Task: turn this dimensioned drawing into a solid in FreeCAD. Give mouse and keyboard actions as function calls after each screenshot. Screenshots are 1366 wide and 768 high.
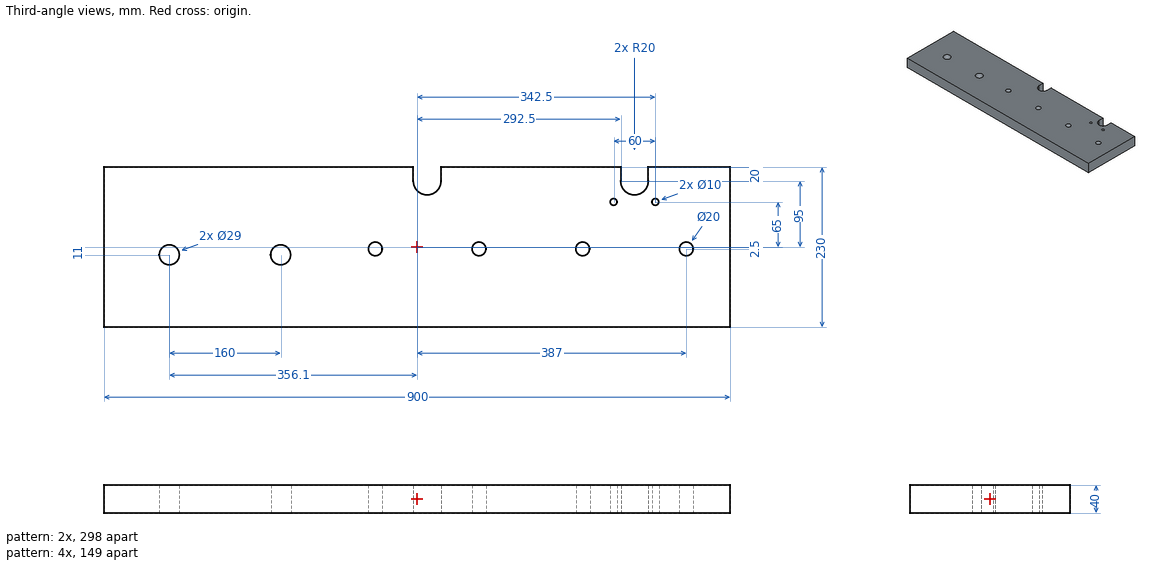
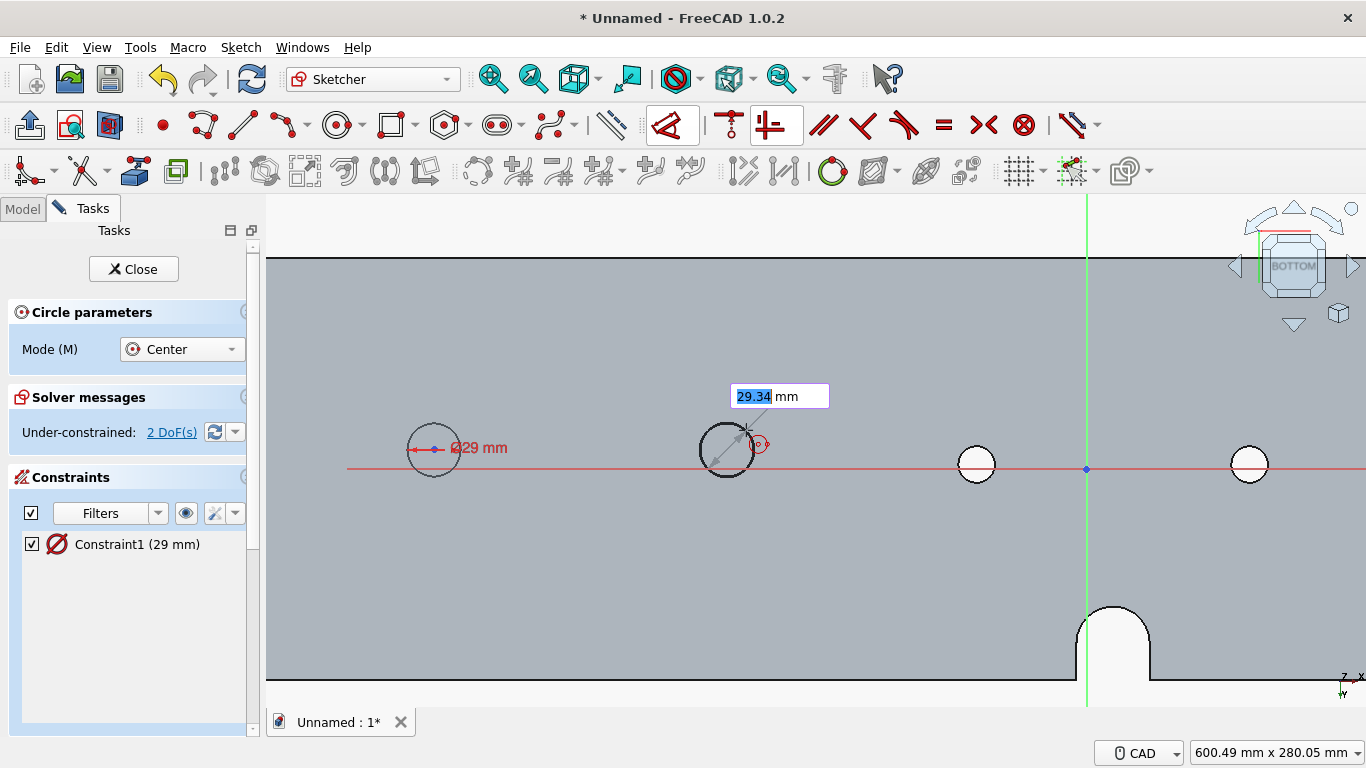
text(29)
key(Return)
key(Escape)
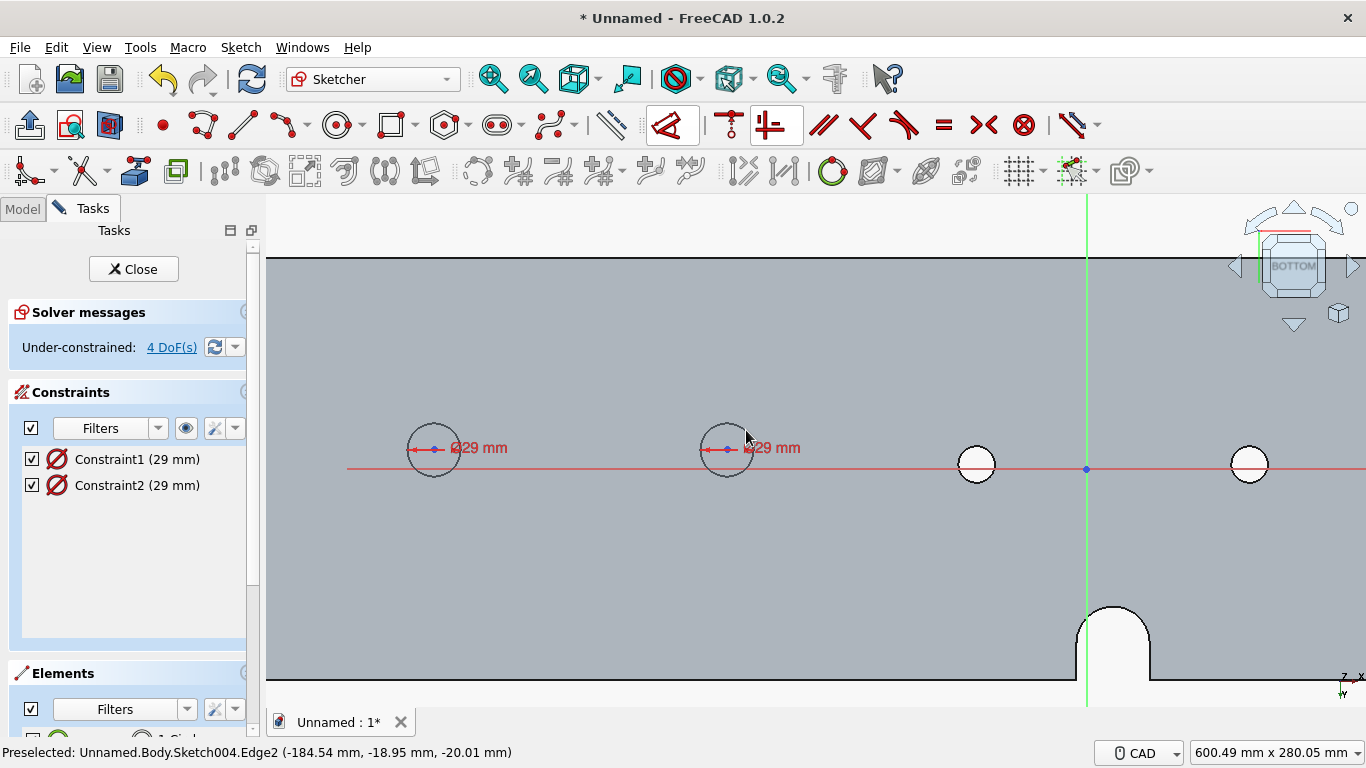
click(434, 450)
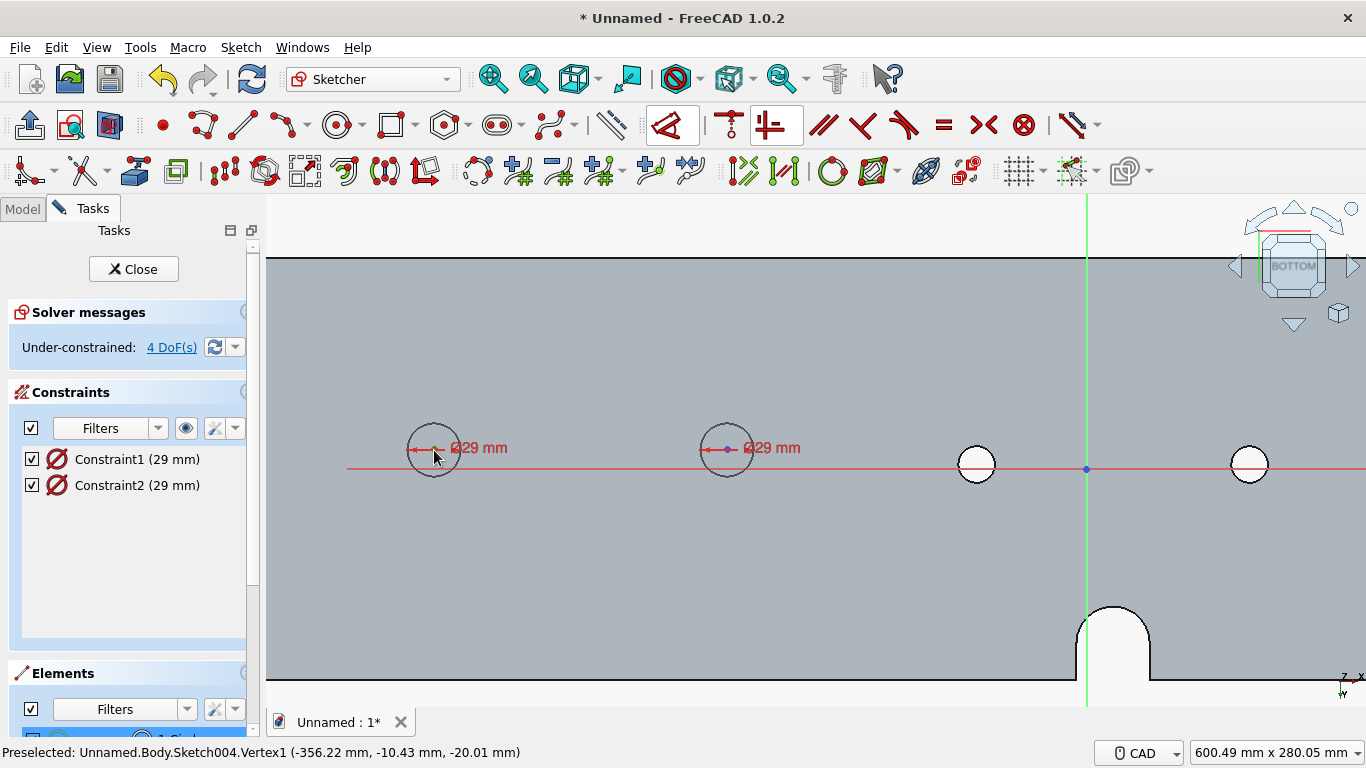
click(727, 450)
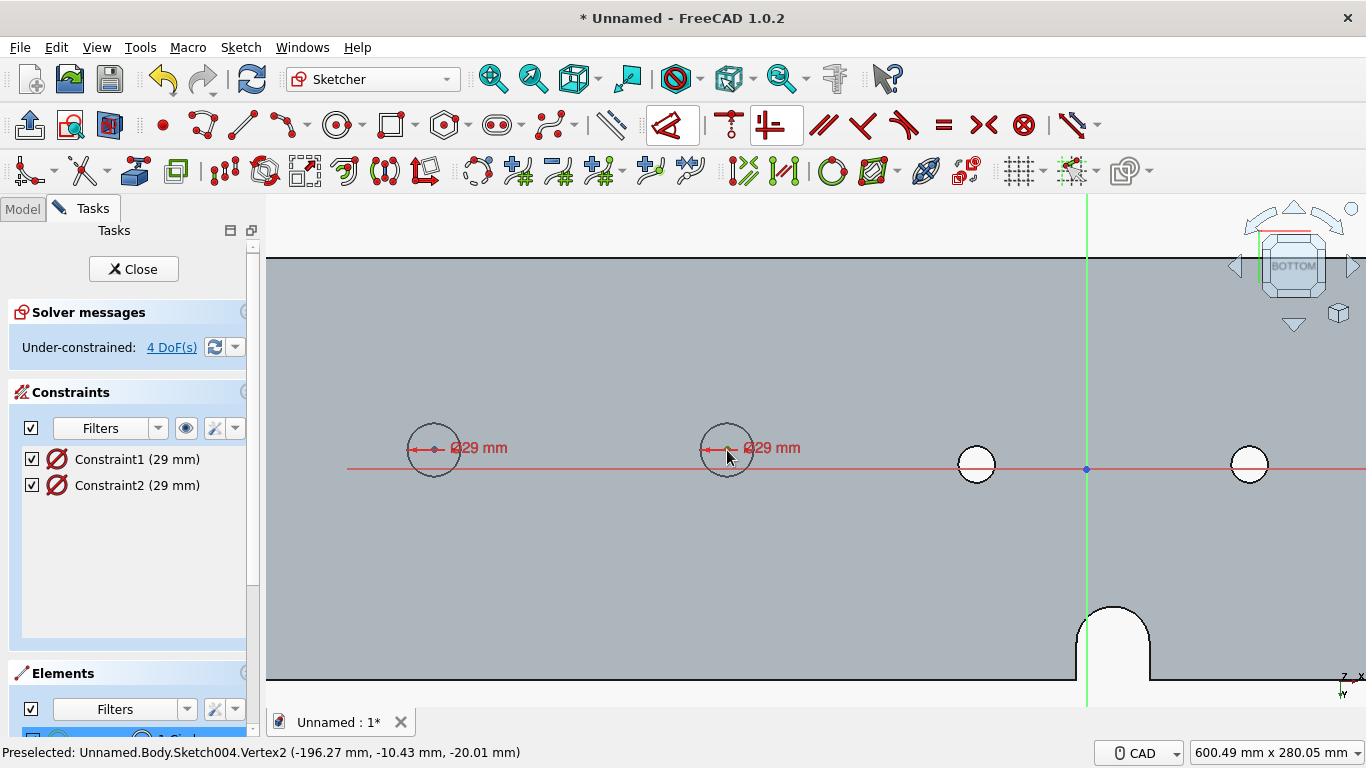
key(h)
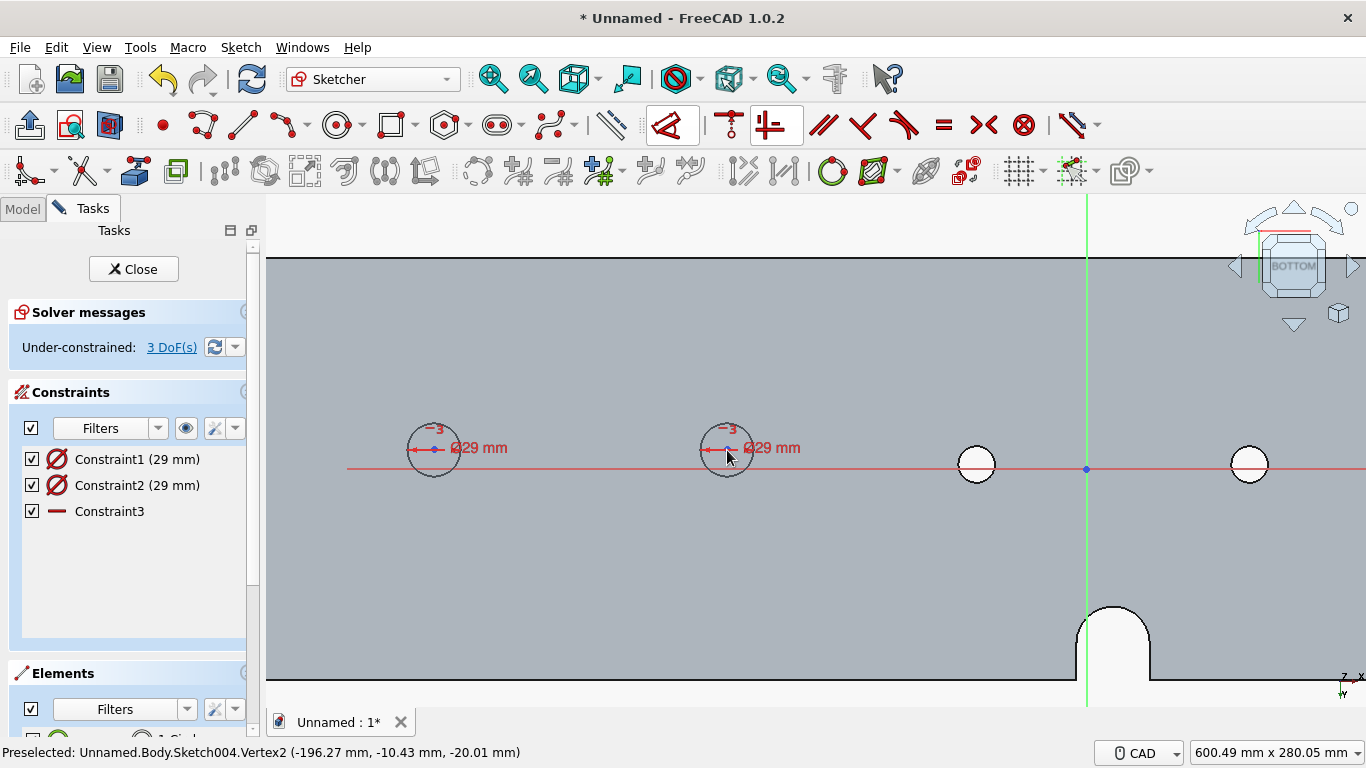
scroll(434, 450, up, 4)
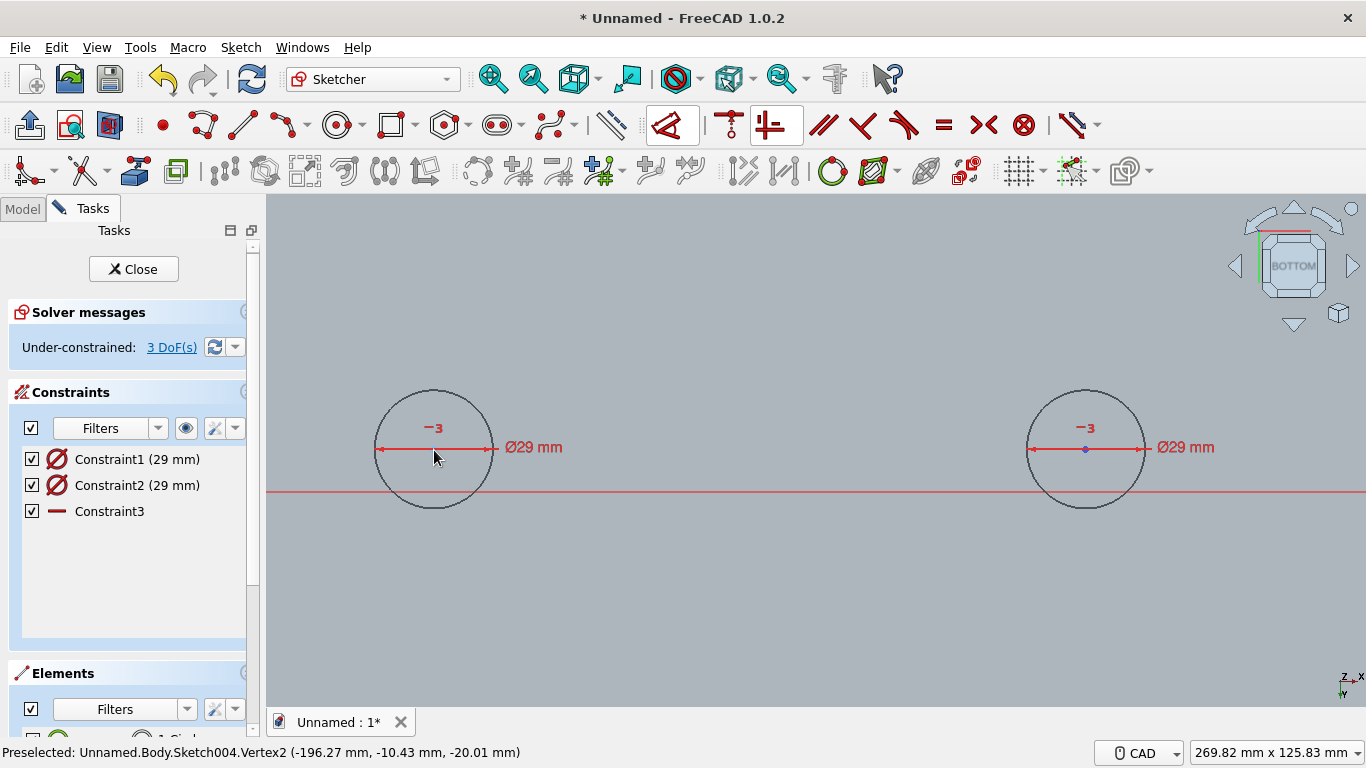
click(434, 449)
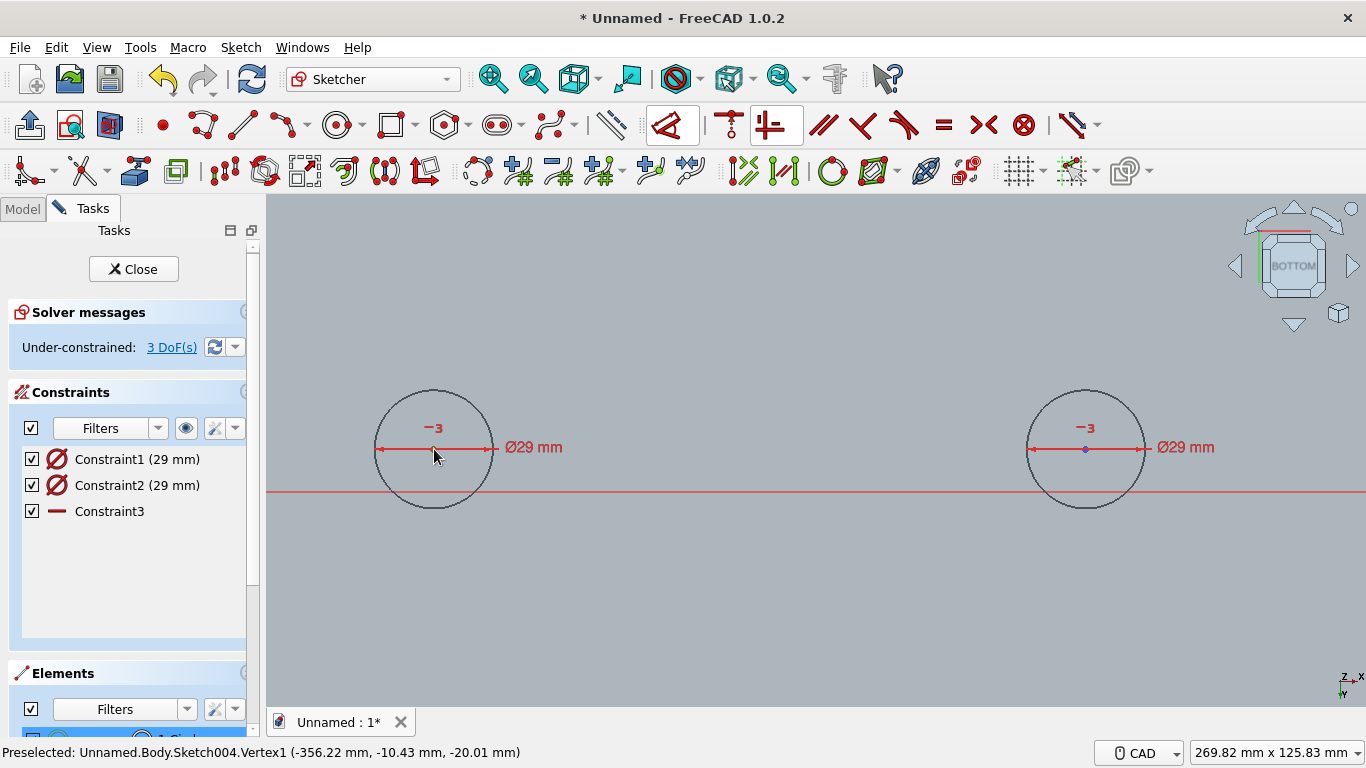
key(i)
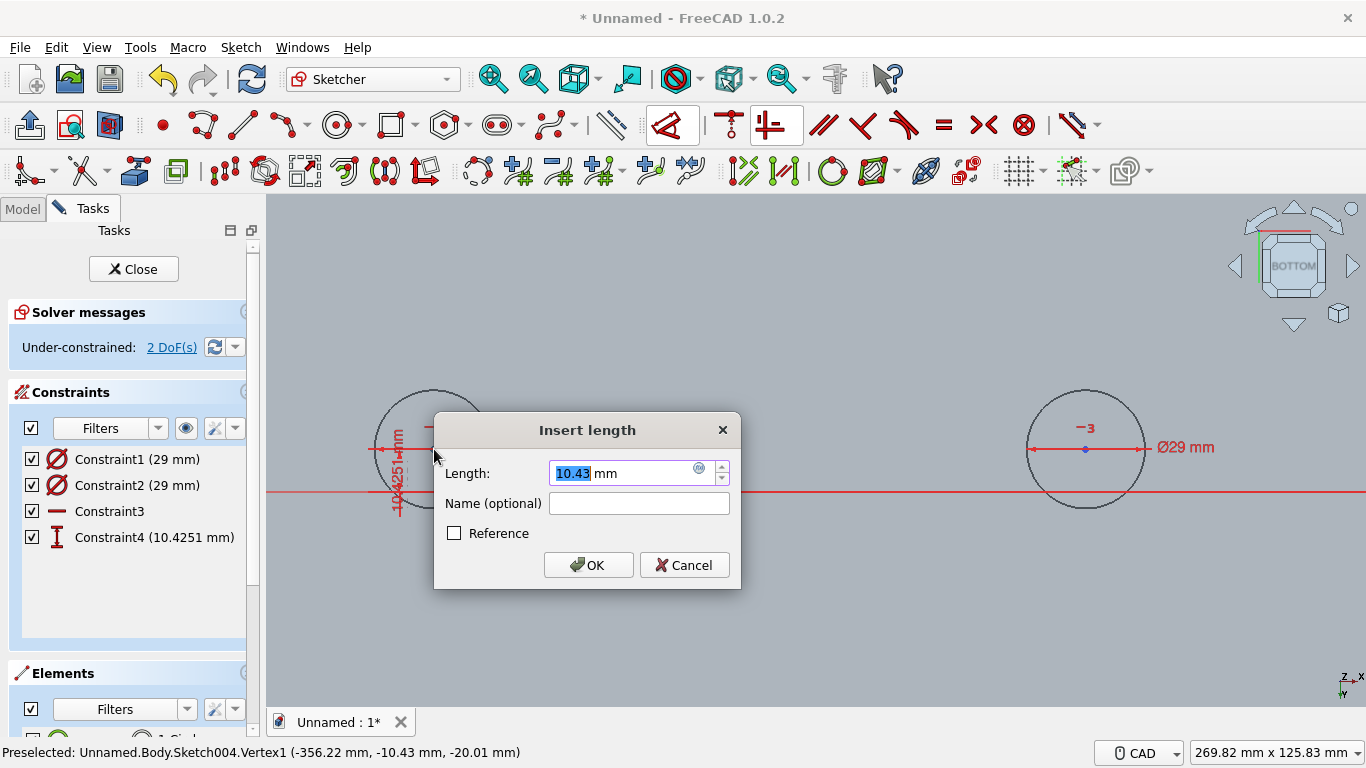
text(11)
key(Return)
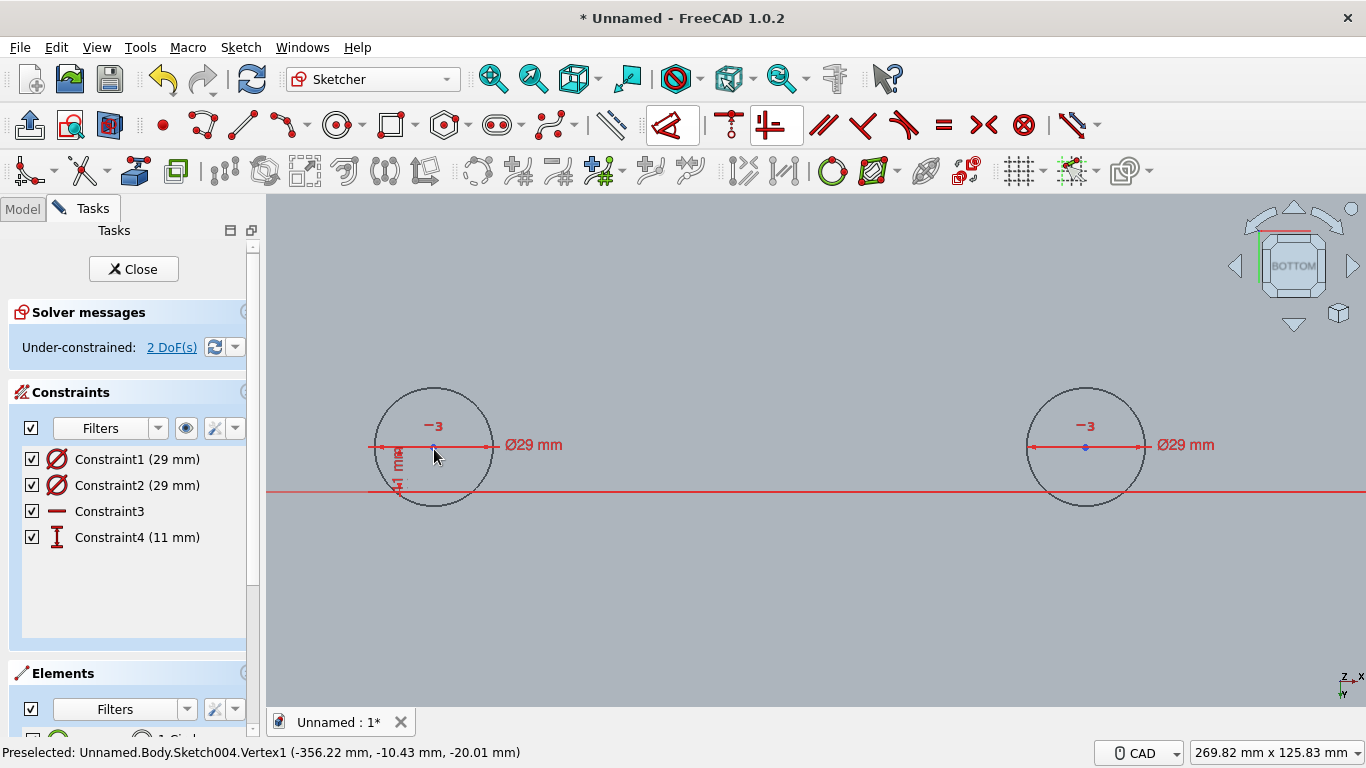
click(434, 447)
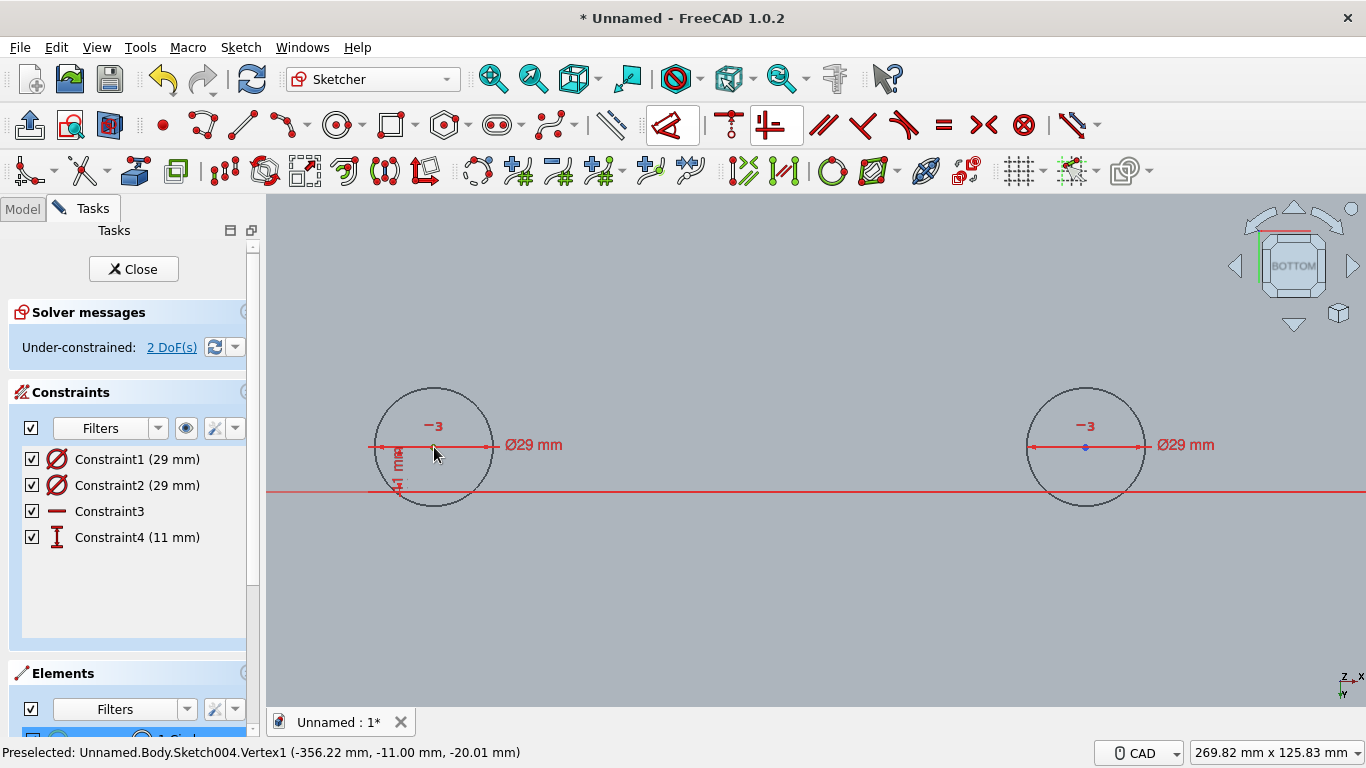
click(1086, 447)